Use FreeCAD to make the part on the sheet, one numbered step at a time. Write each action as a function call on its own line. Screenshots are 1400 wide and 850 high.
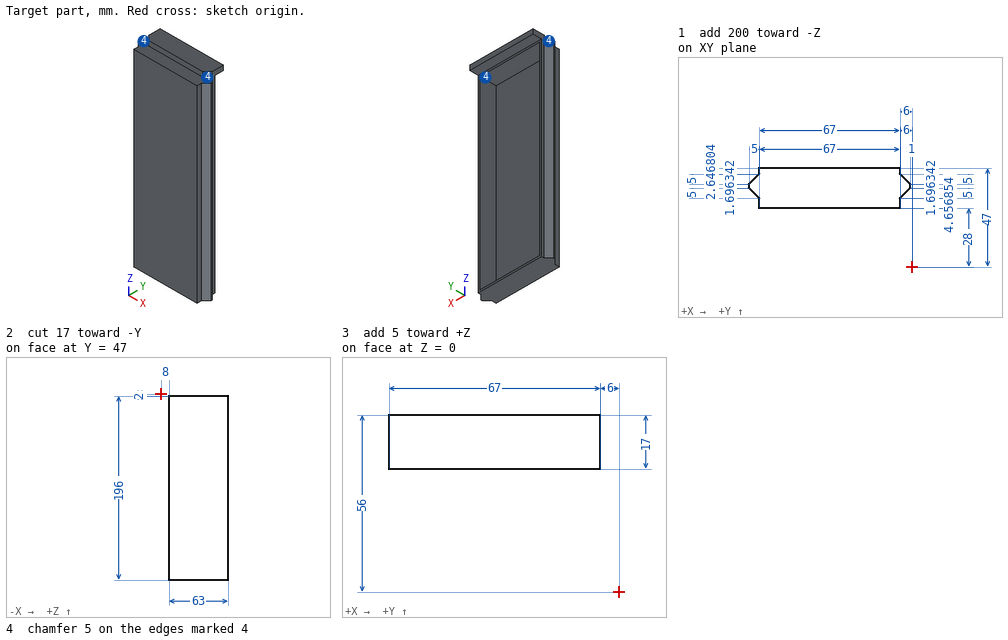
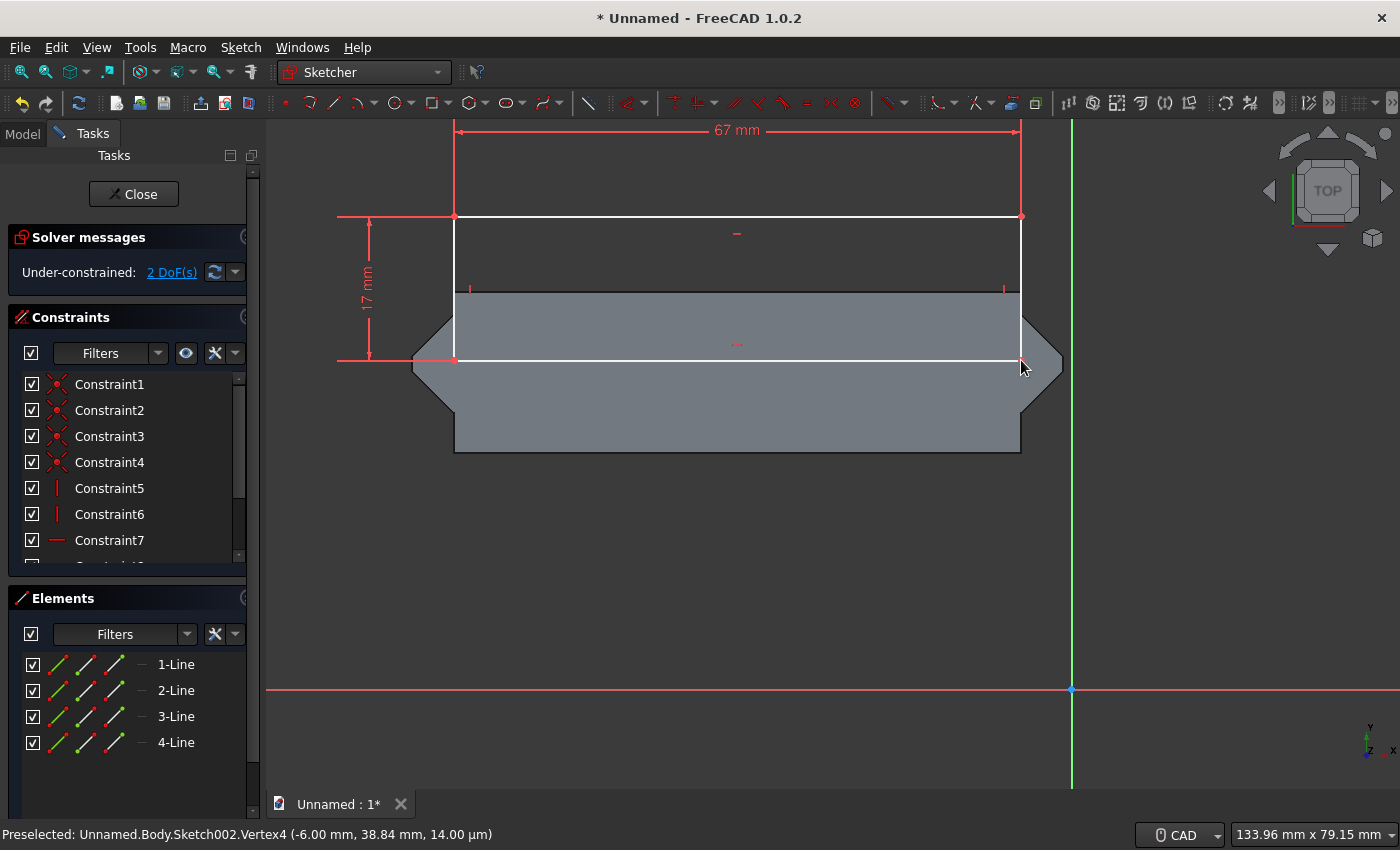
click(628, 104)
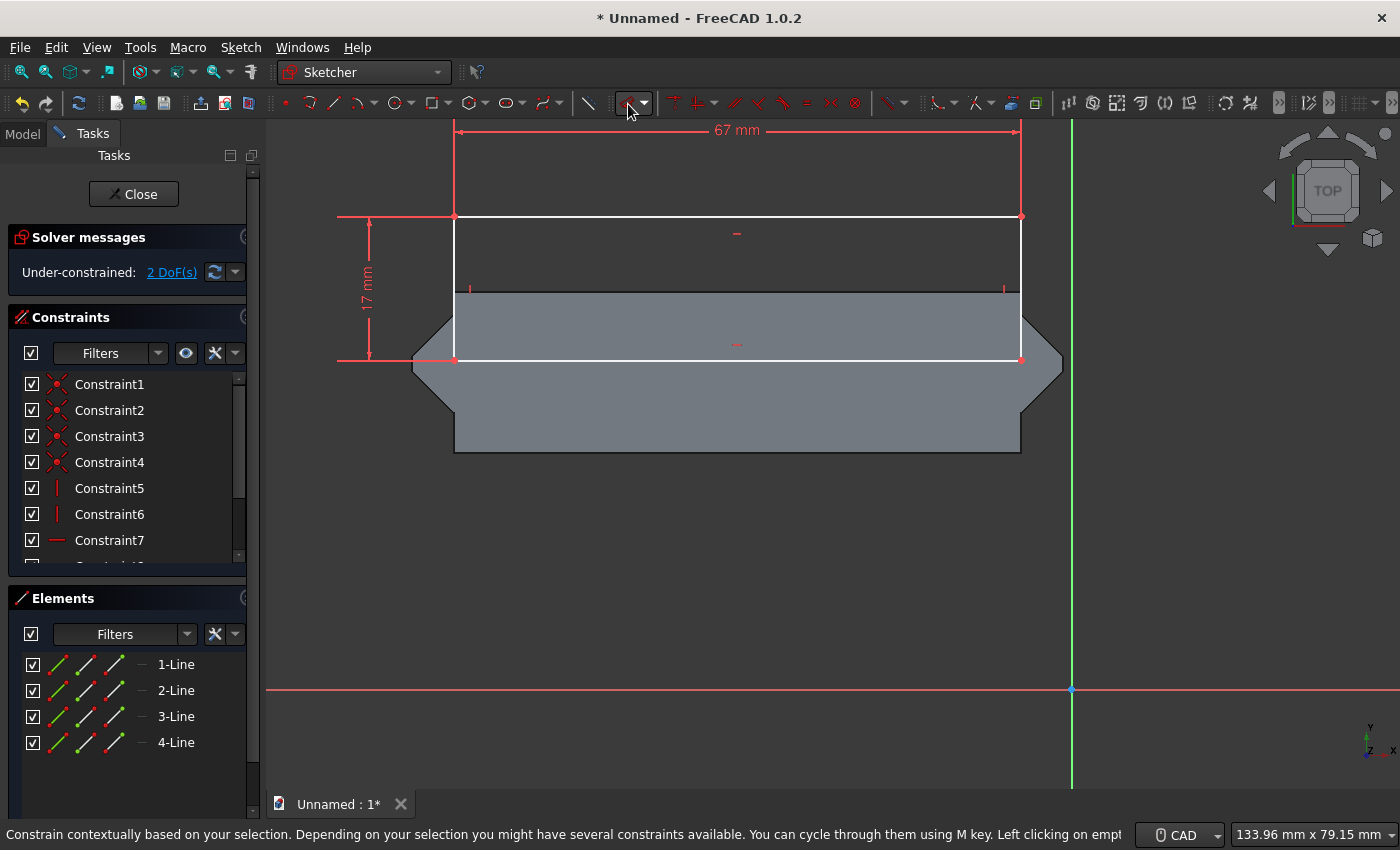
click(1021, 361)
click(1047, 724)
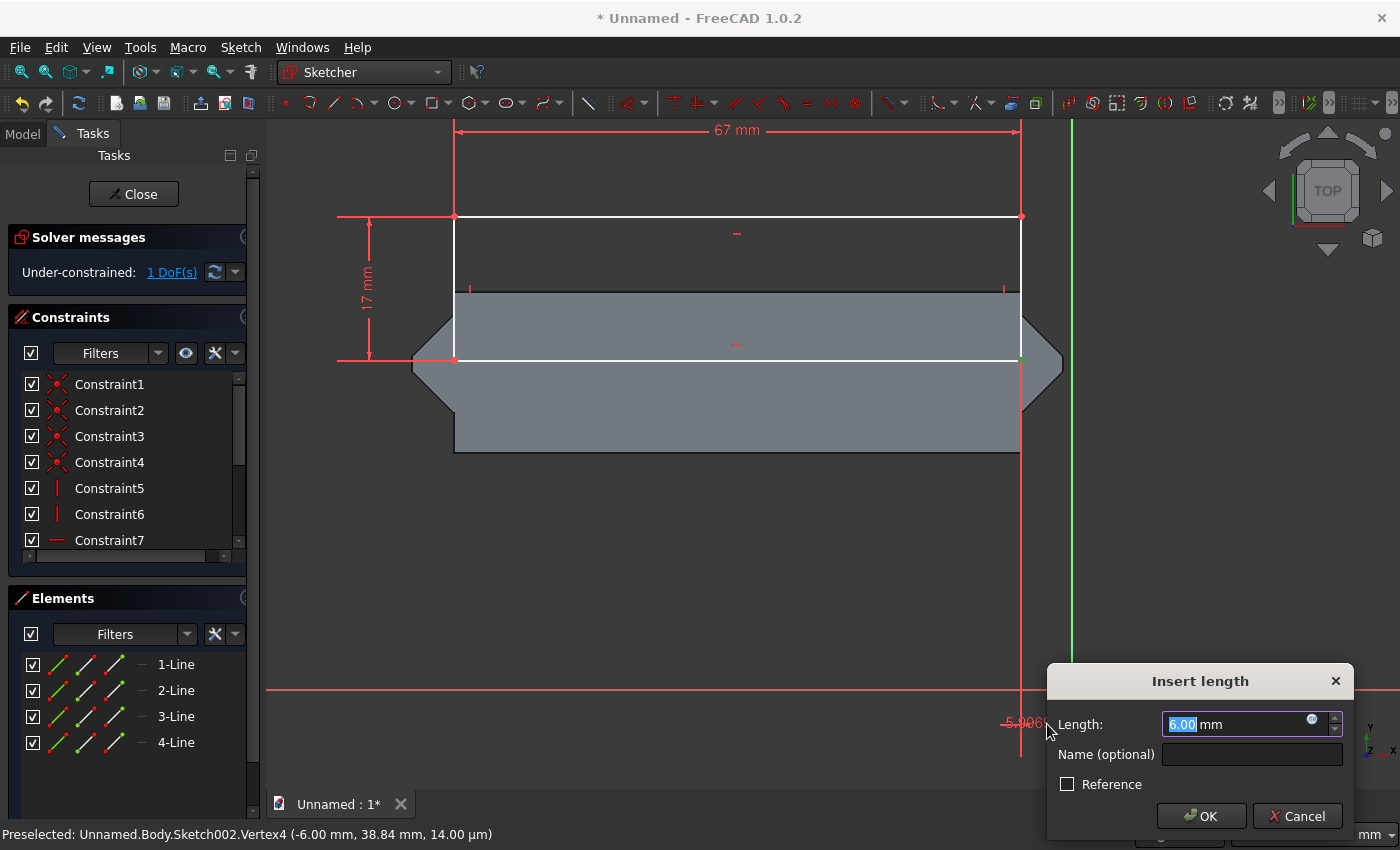
text(6)
key(Return)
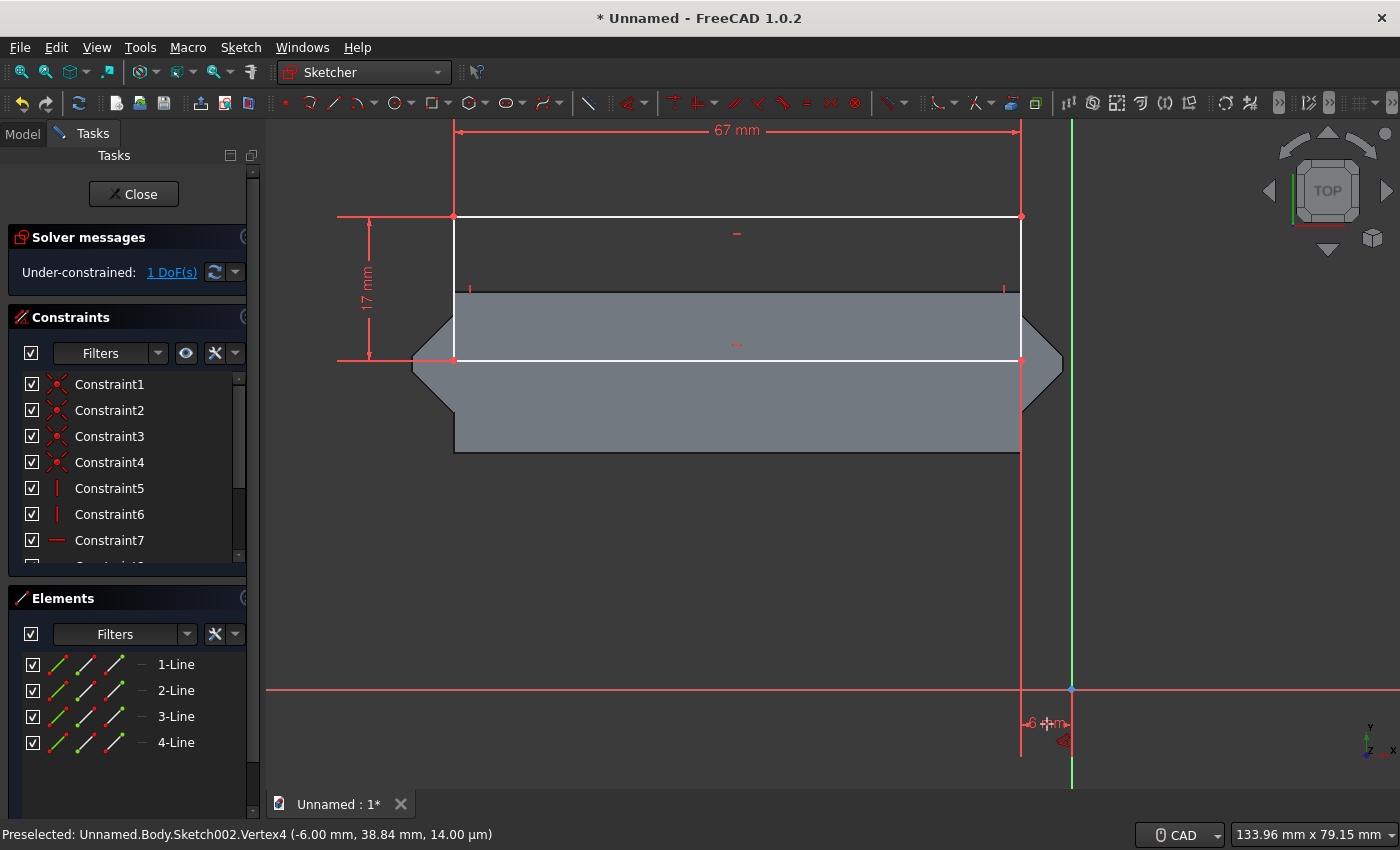
click(454, 217)
click(1106, 453)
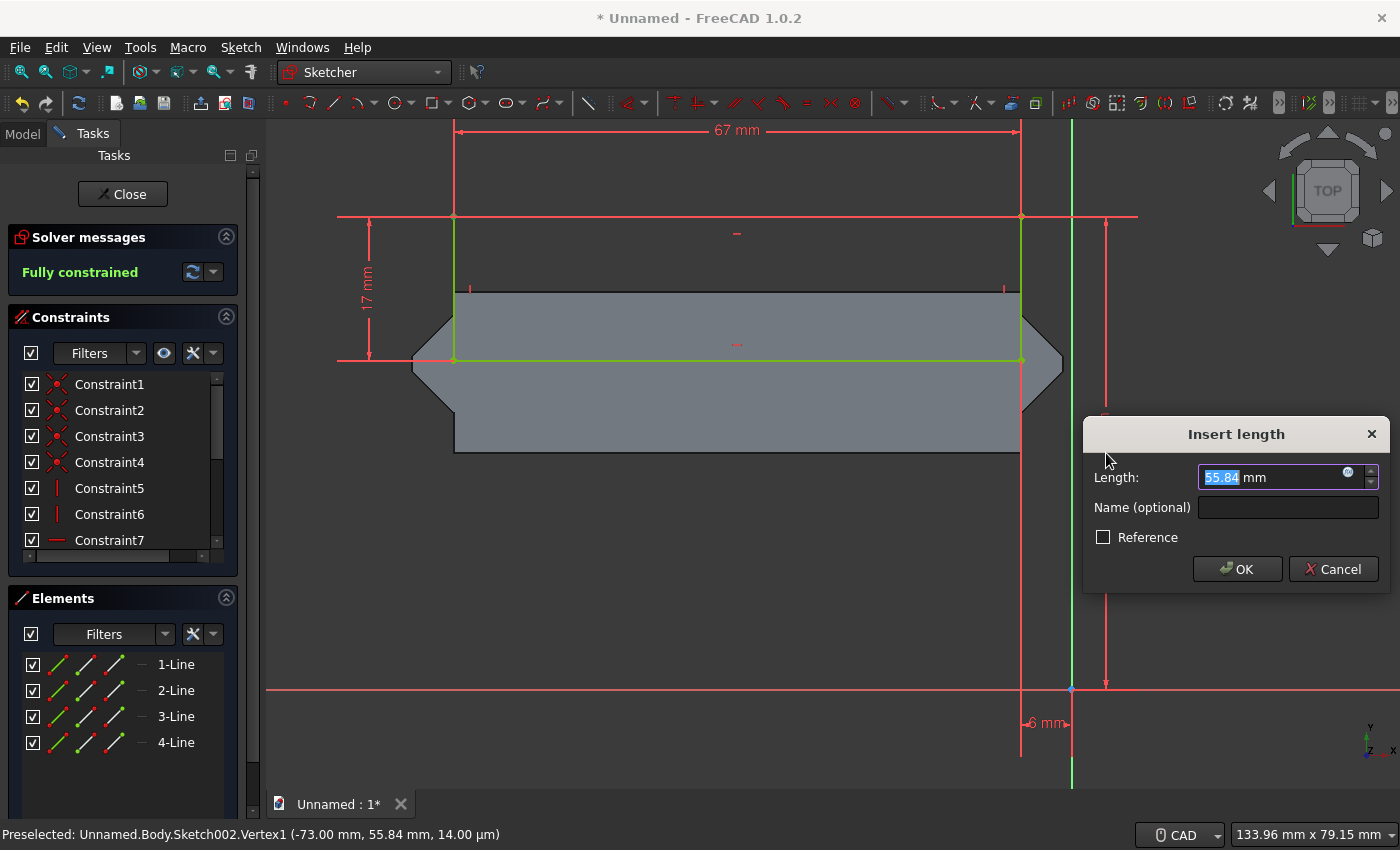
text(56)
key(Return)
key(Escape)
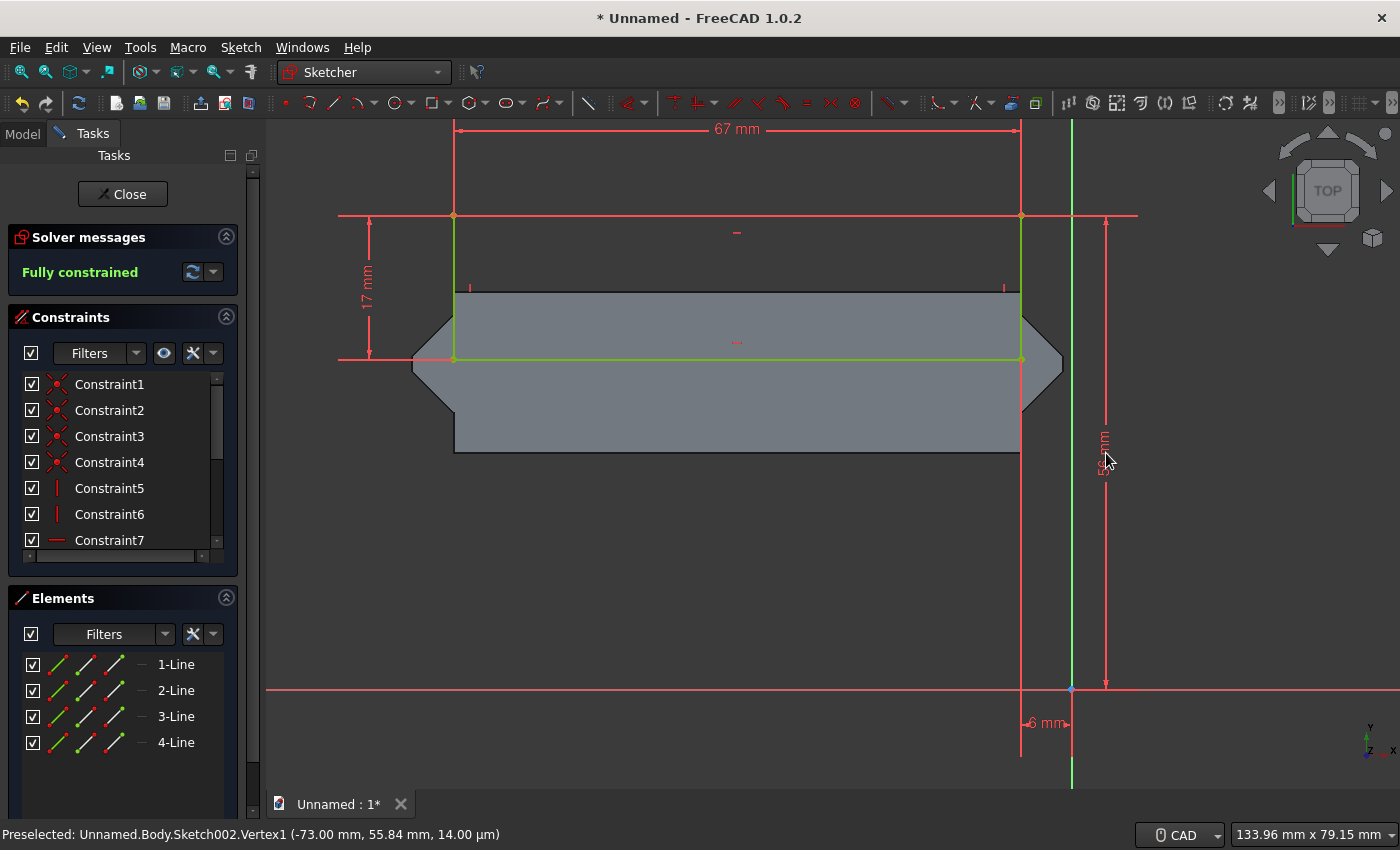
click(123, 194)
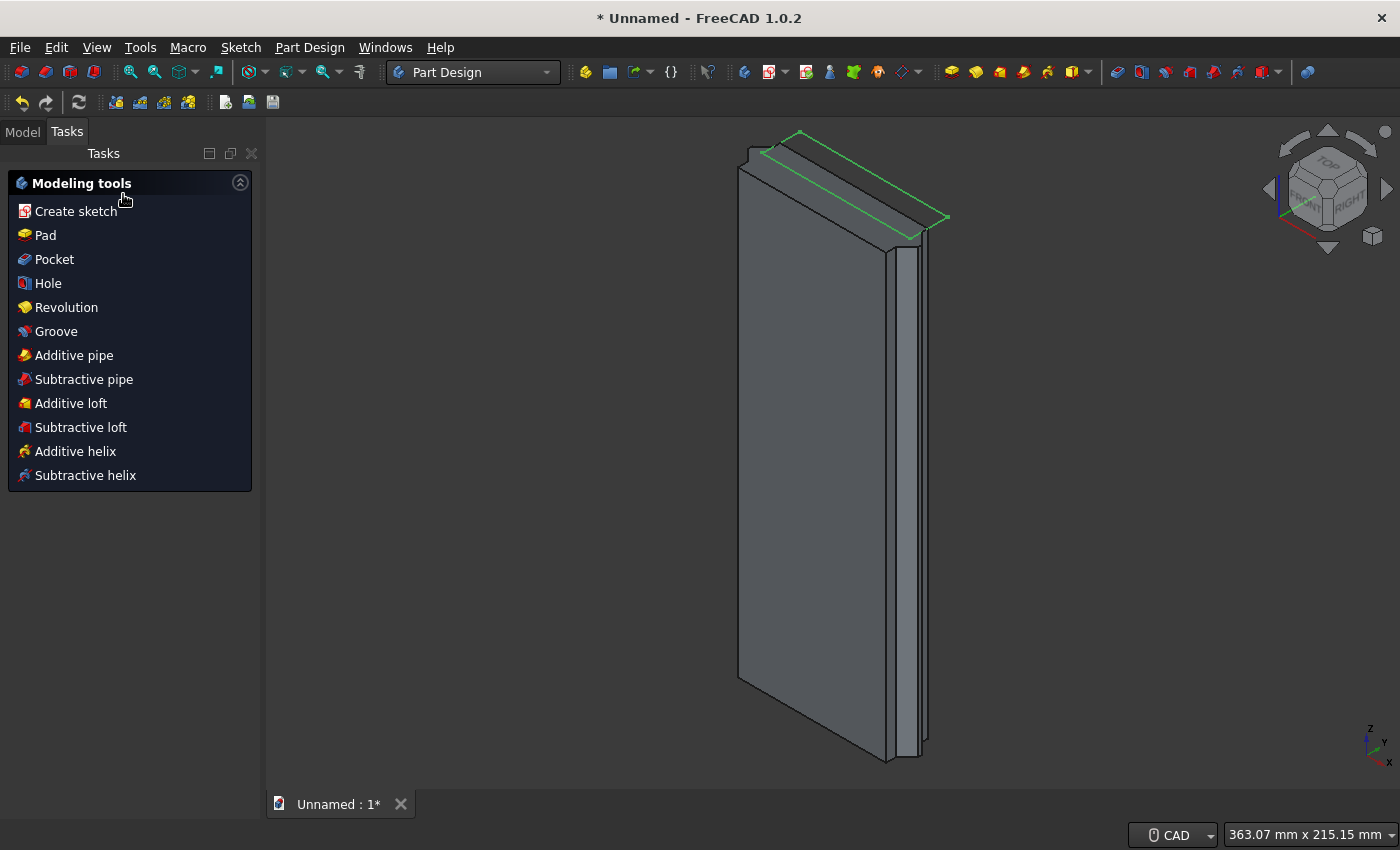
click(952, 72)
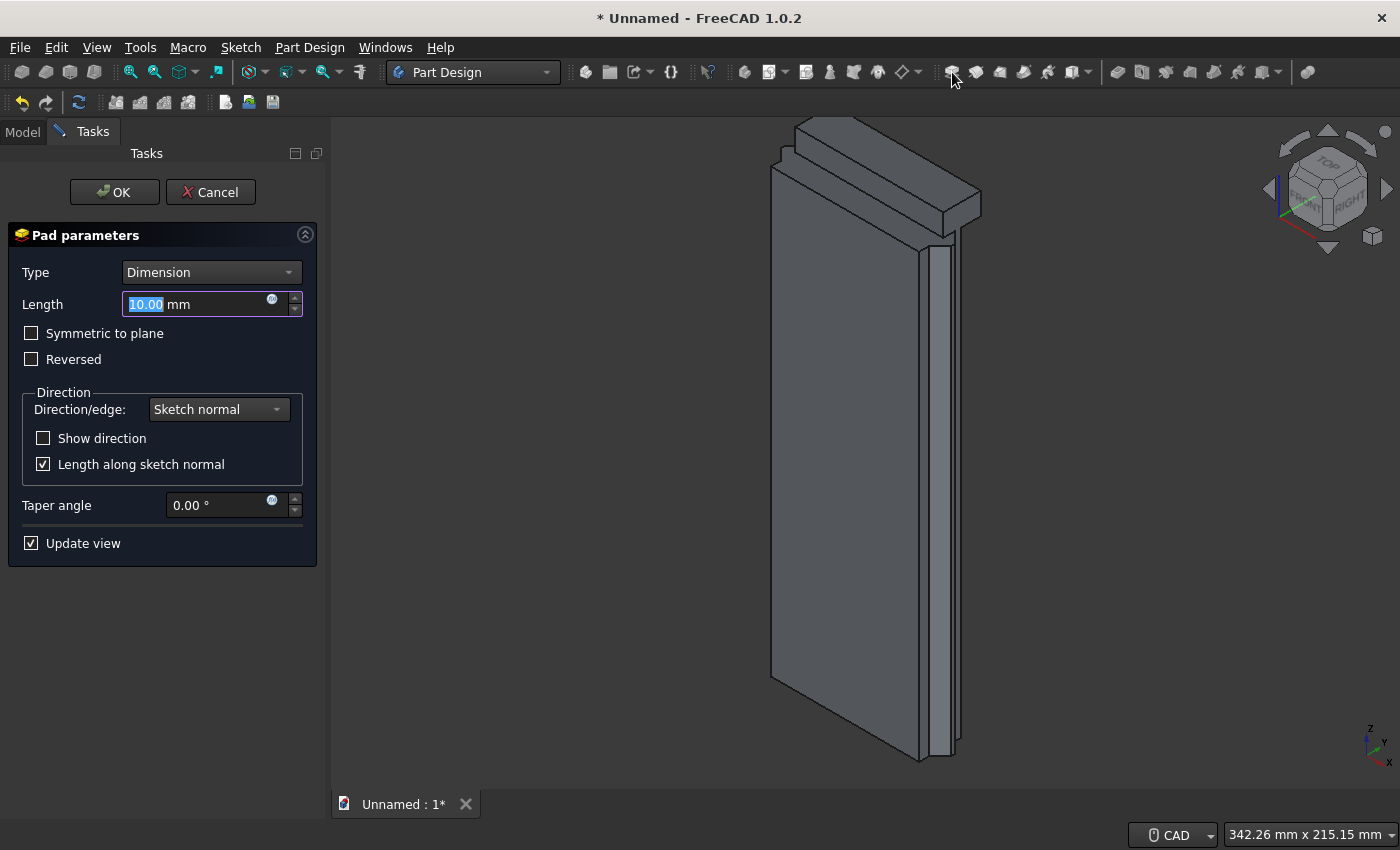
text(5)
key(Tab)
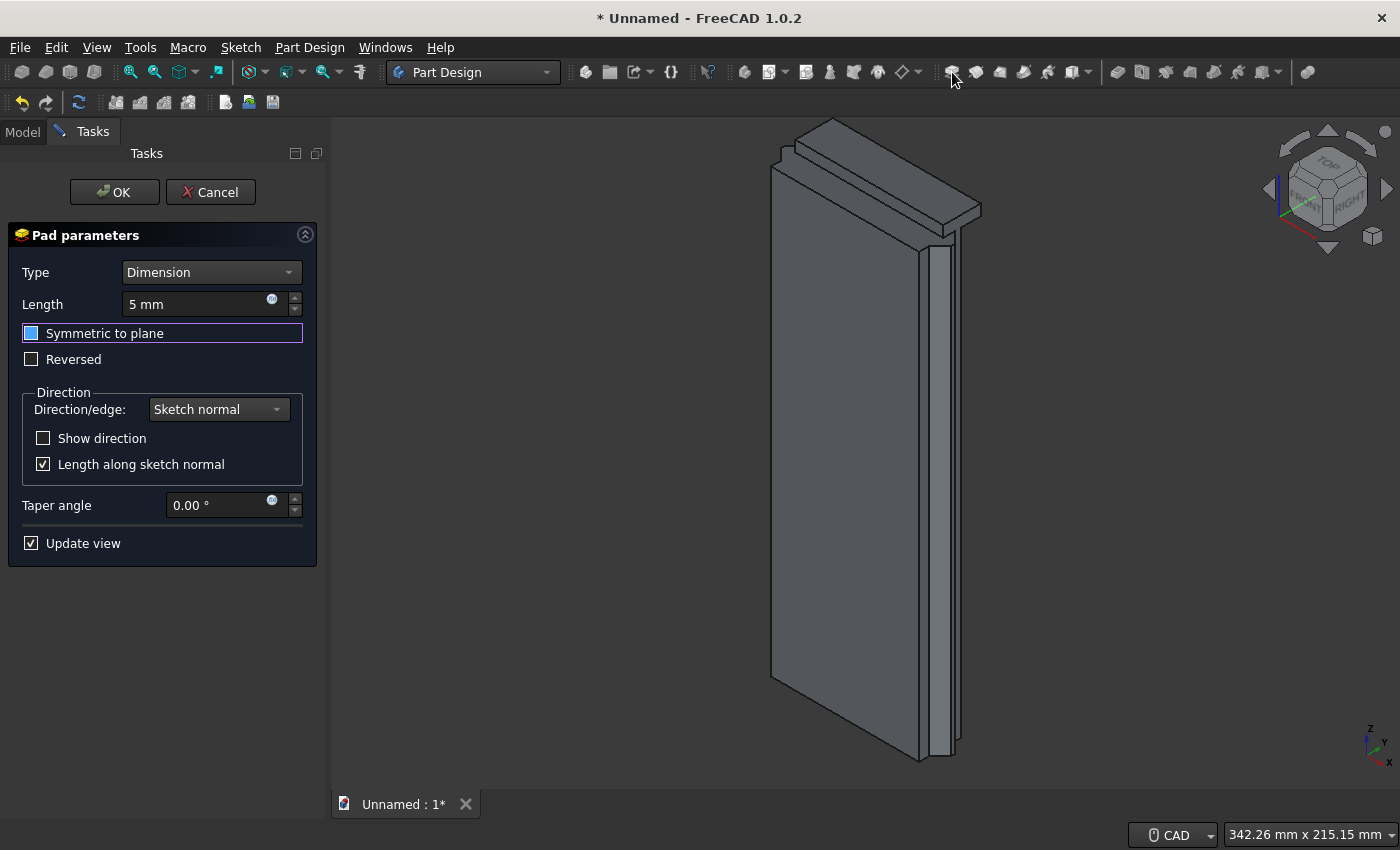
click(115, 192)